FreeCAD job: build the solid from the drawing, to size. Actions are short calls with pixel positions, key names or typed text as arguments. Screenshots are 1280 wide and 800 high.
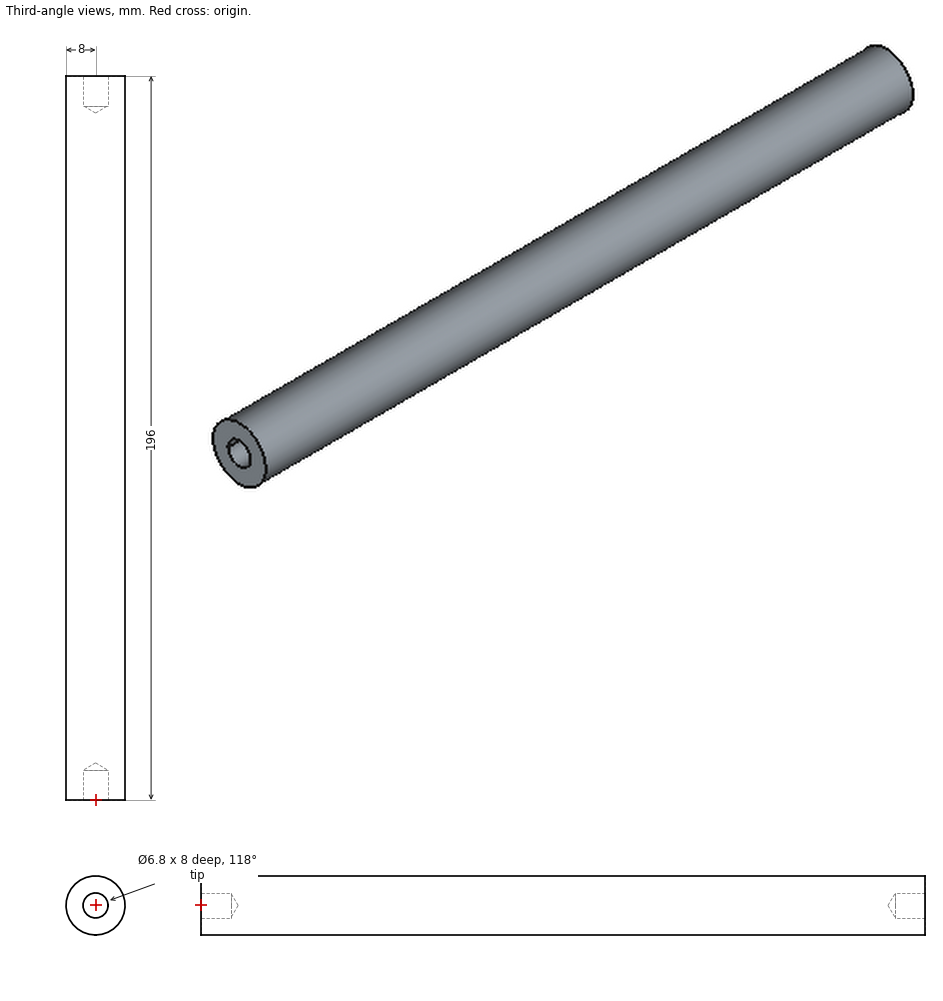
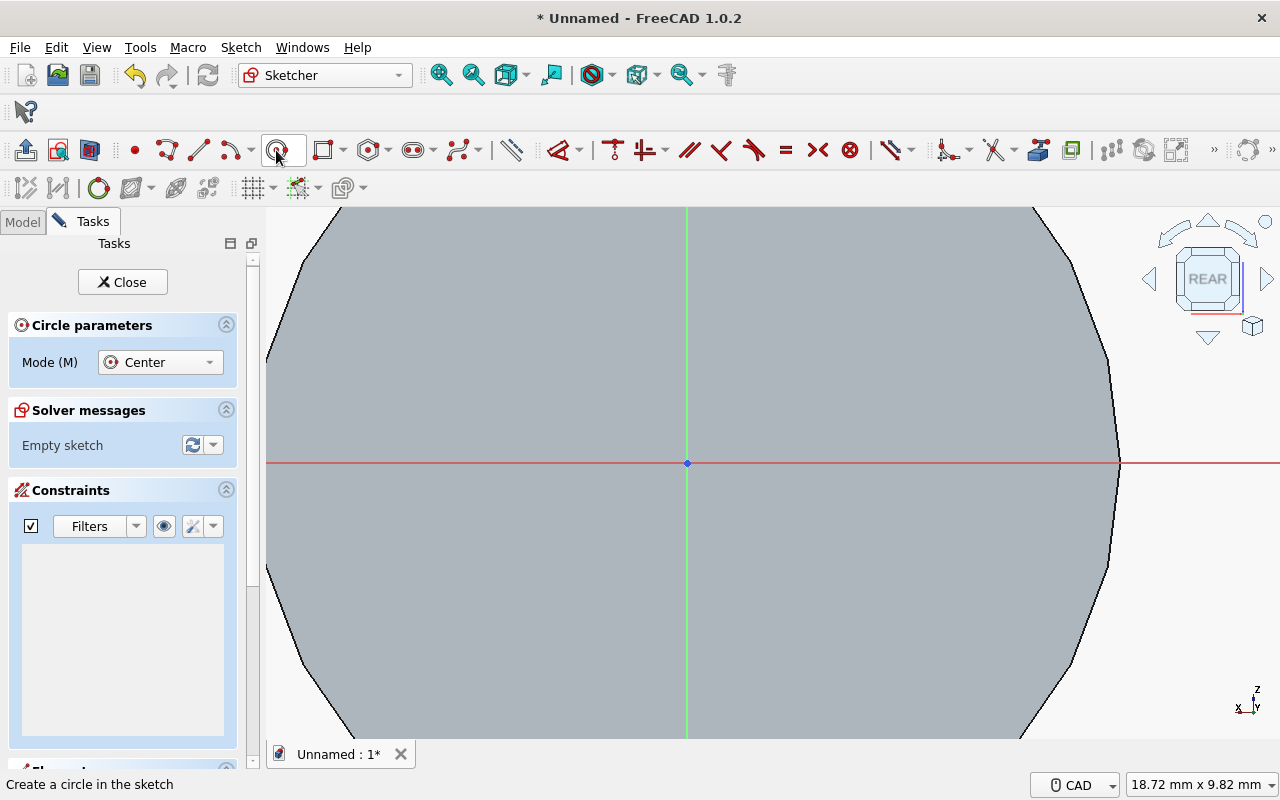
click(687, 463)
move(817, 333)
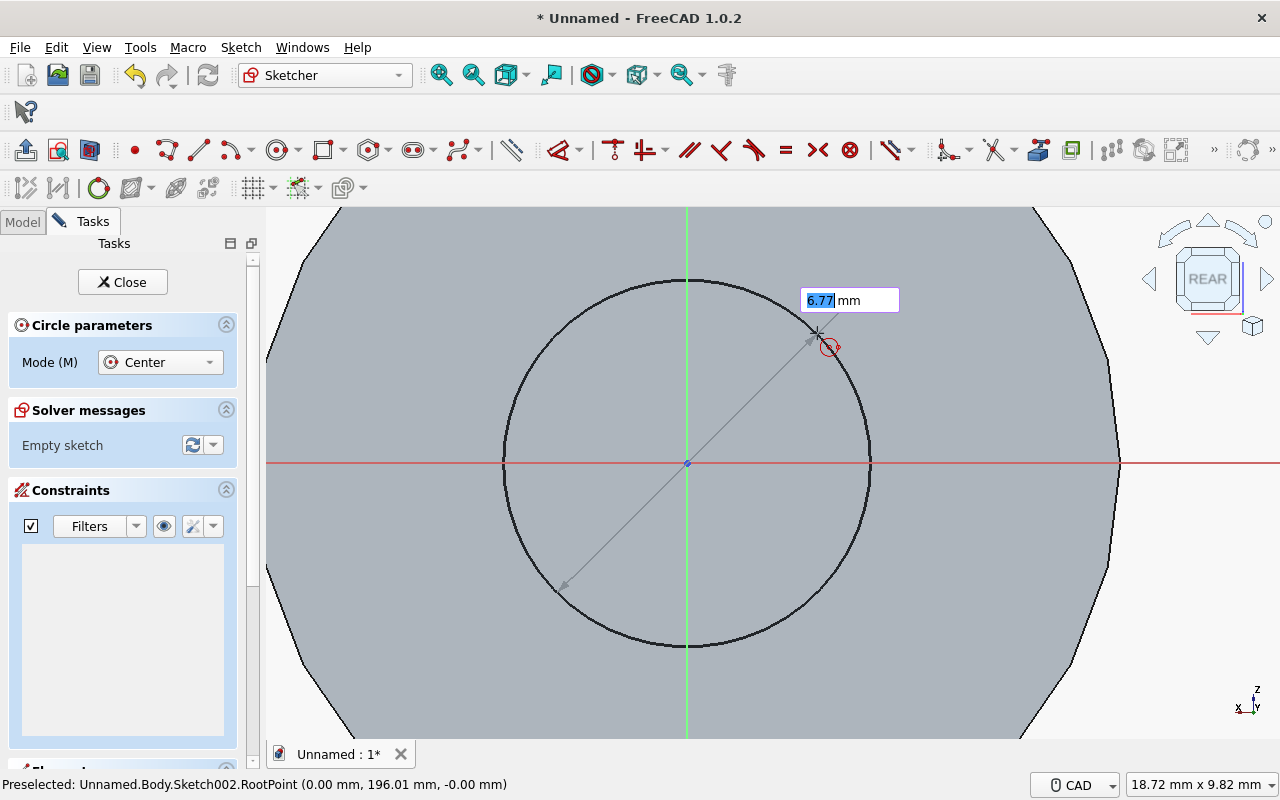
text(6.8)
key(Return)
key(Escape)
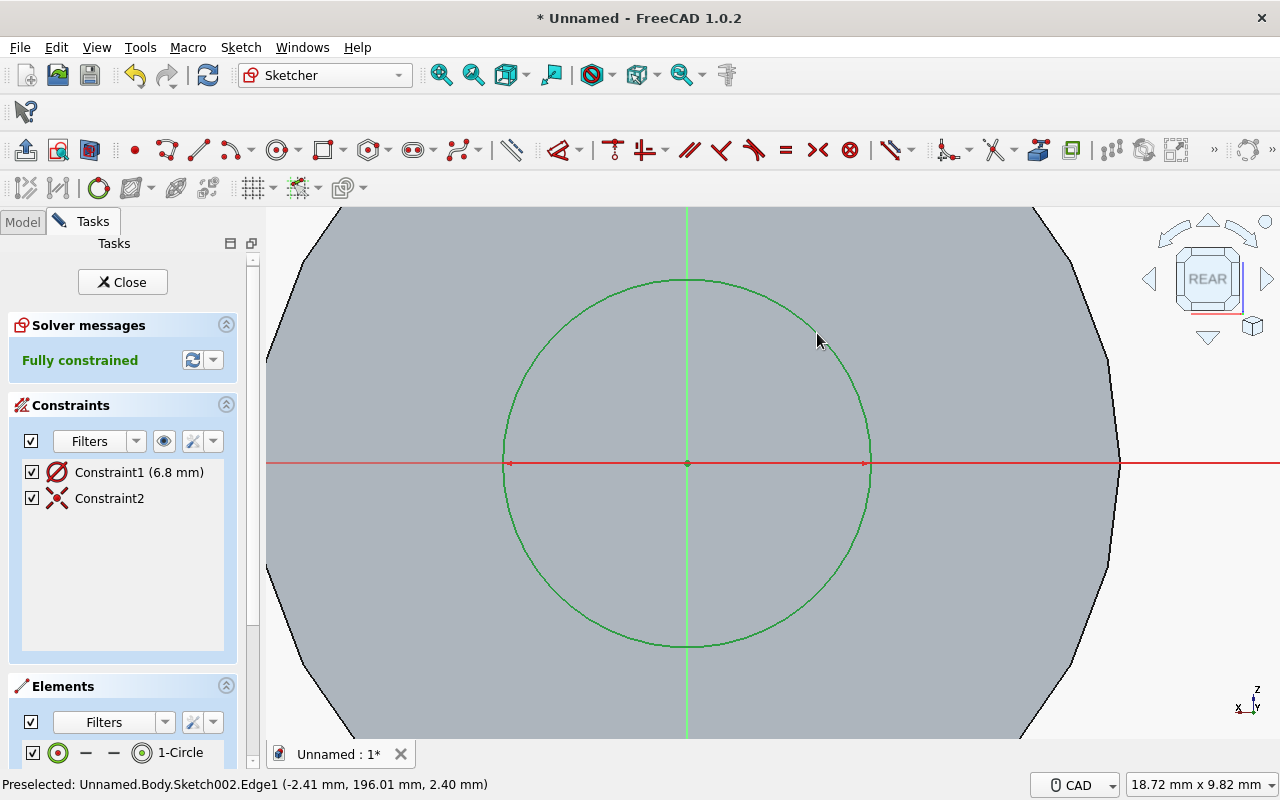
click(123, 282)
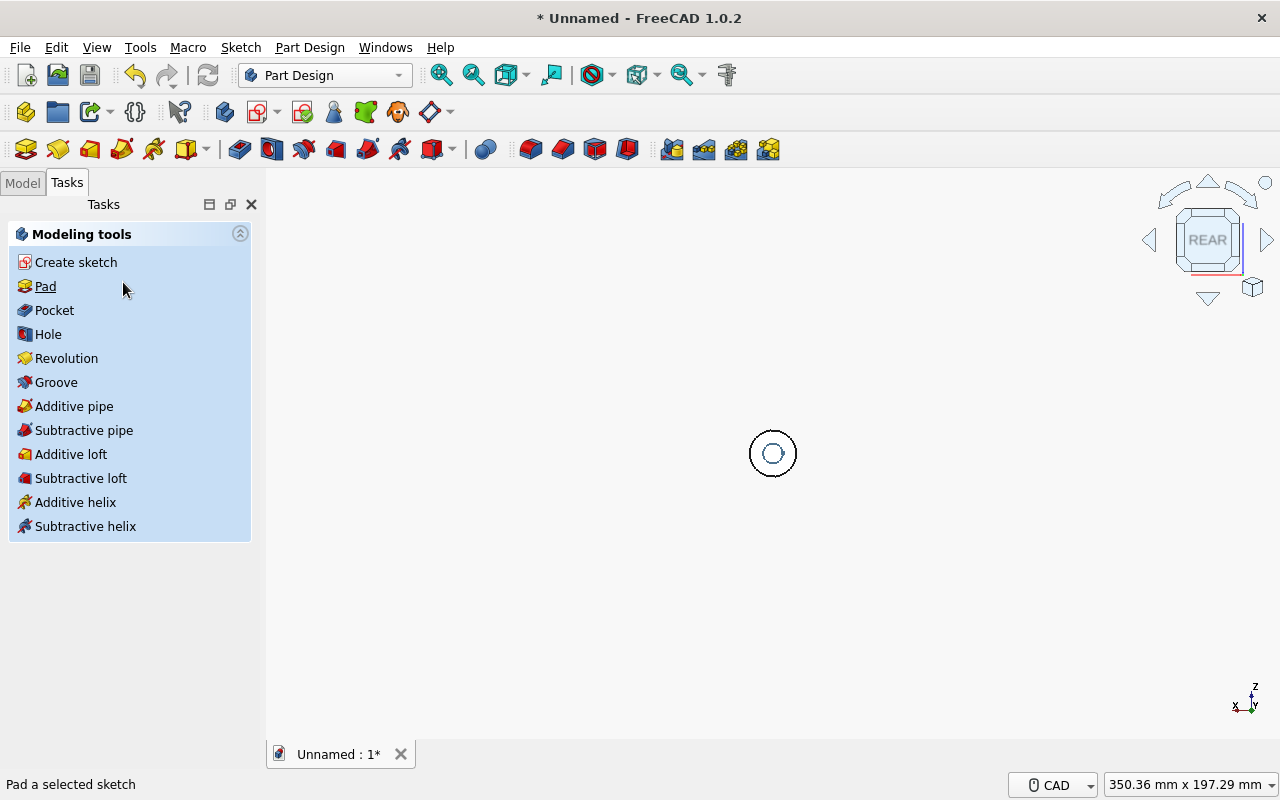
click(272, 150)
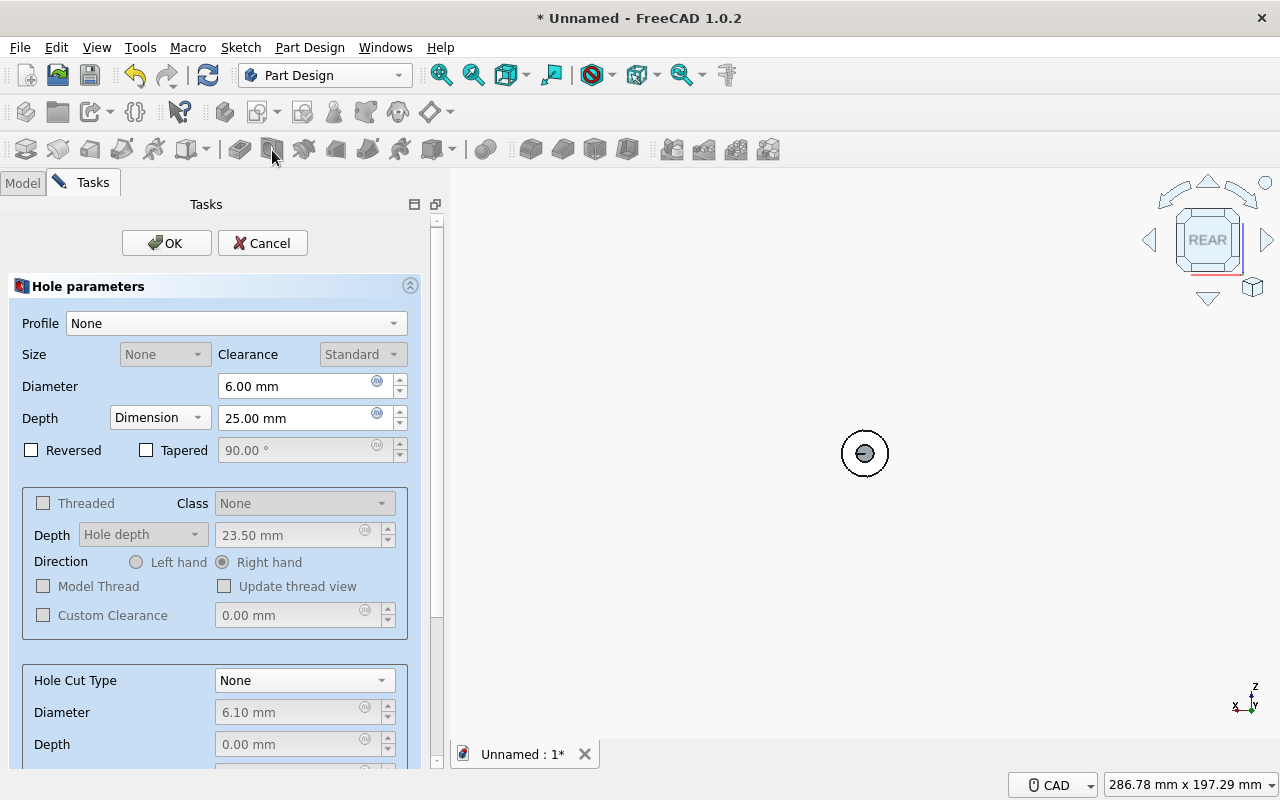
triple_click(305, 386)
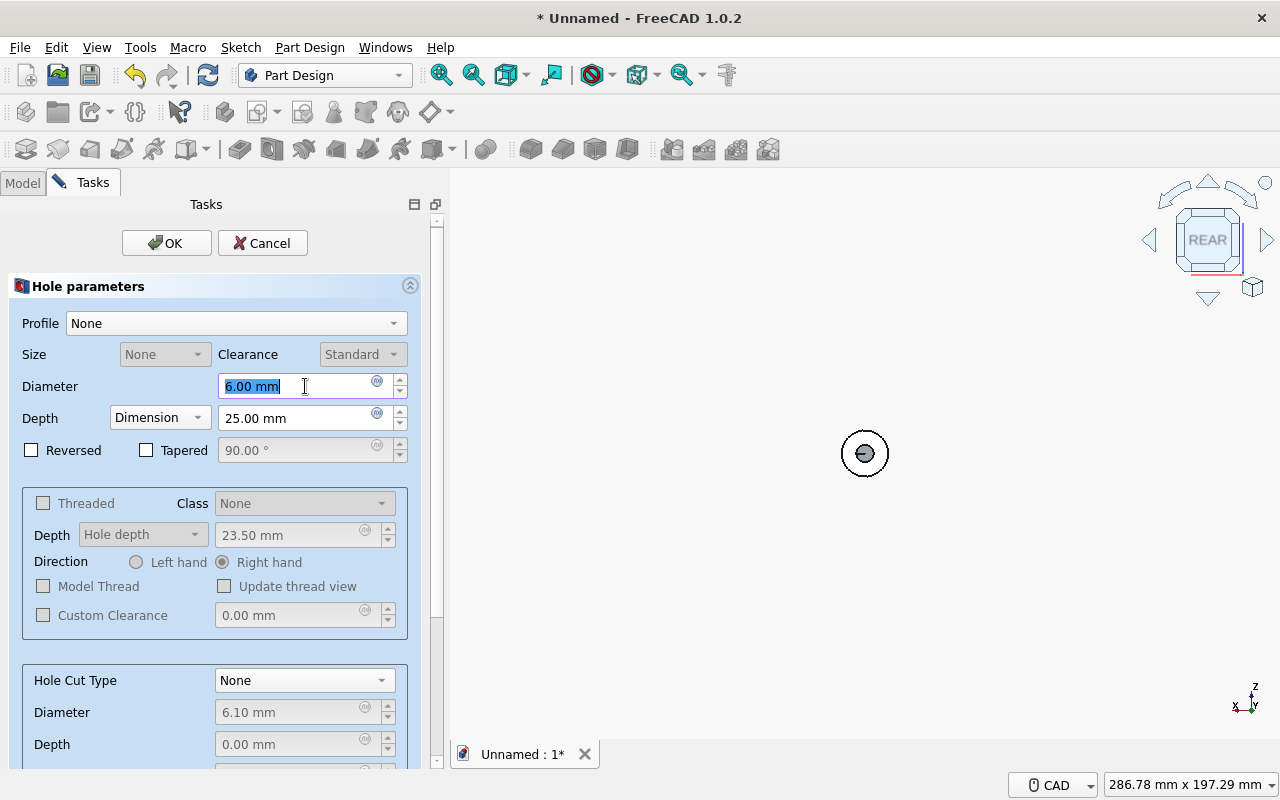
text(6.8)
key(Tab)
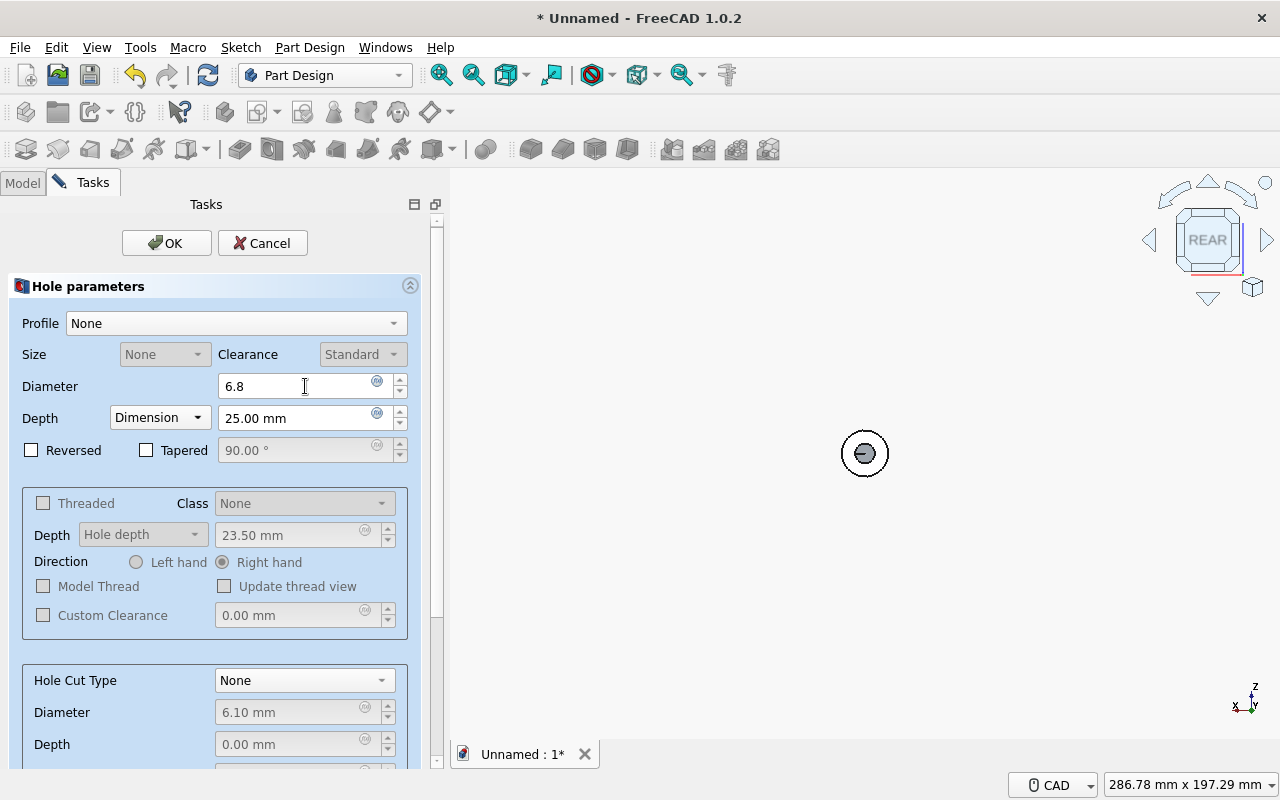
triple_click(305, 418)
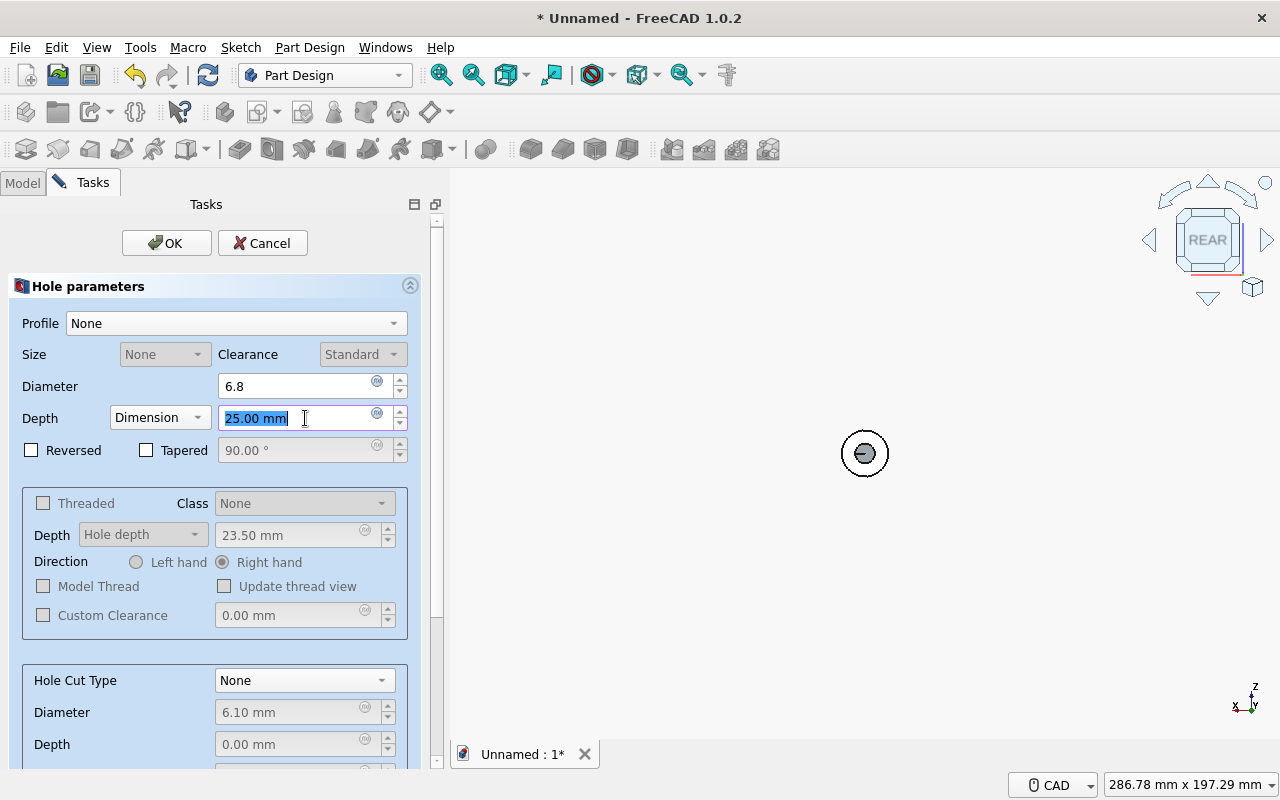
text(8)
key(Tab)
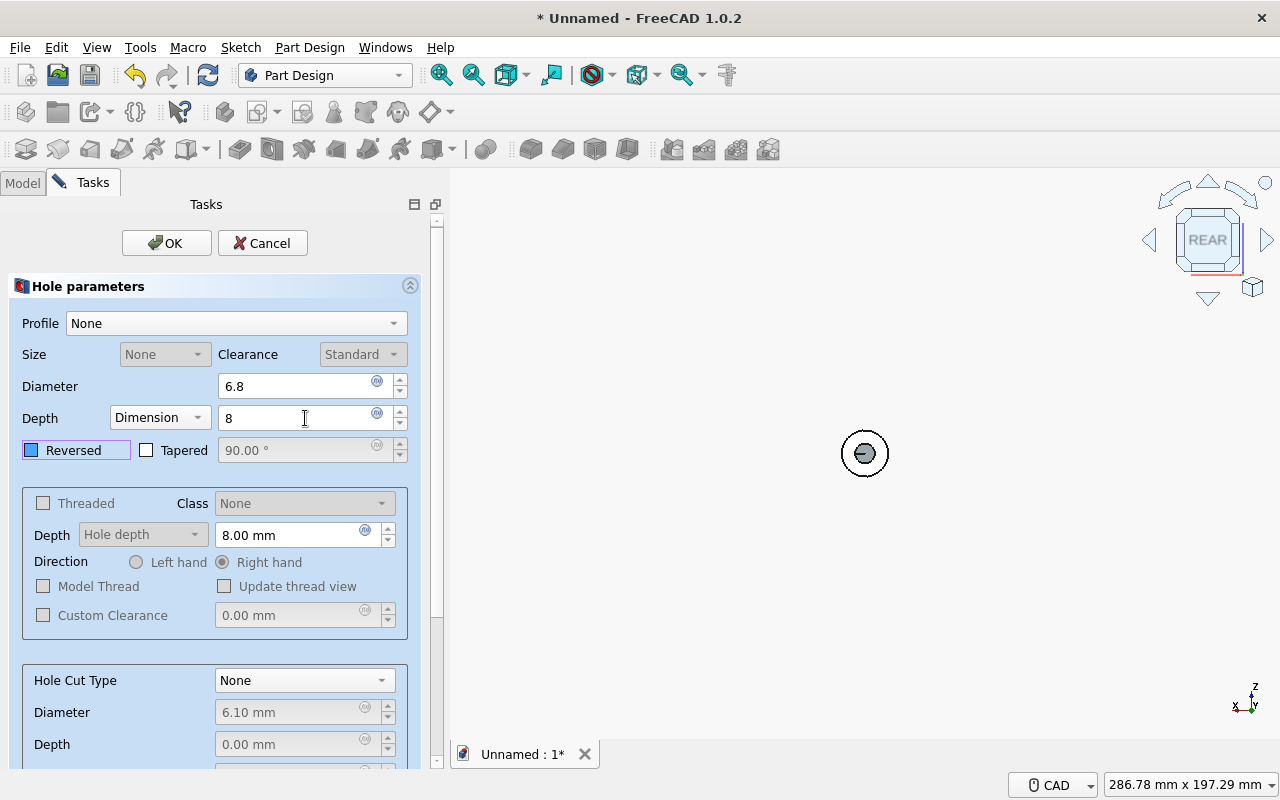
click(167, 243)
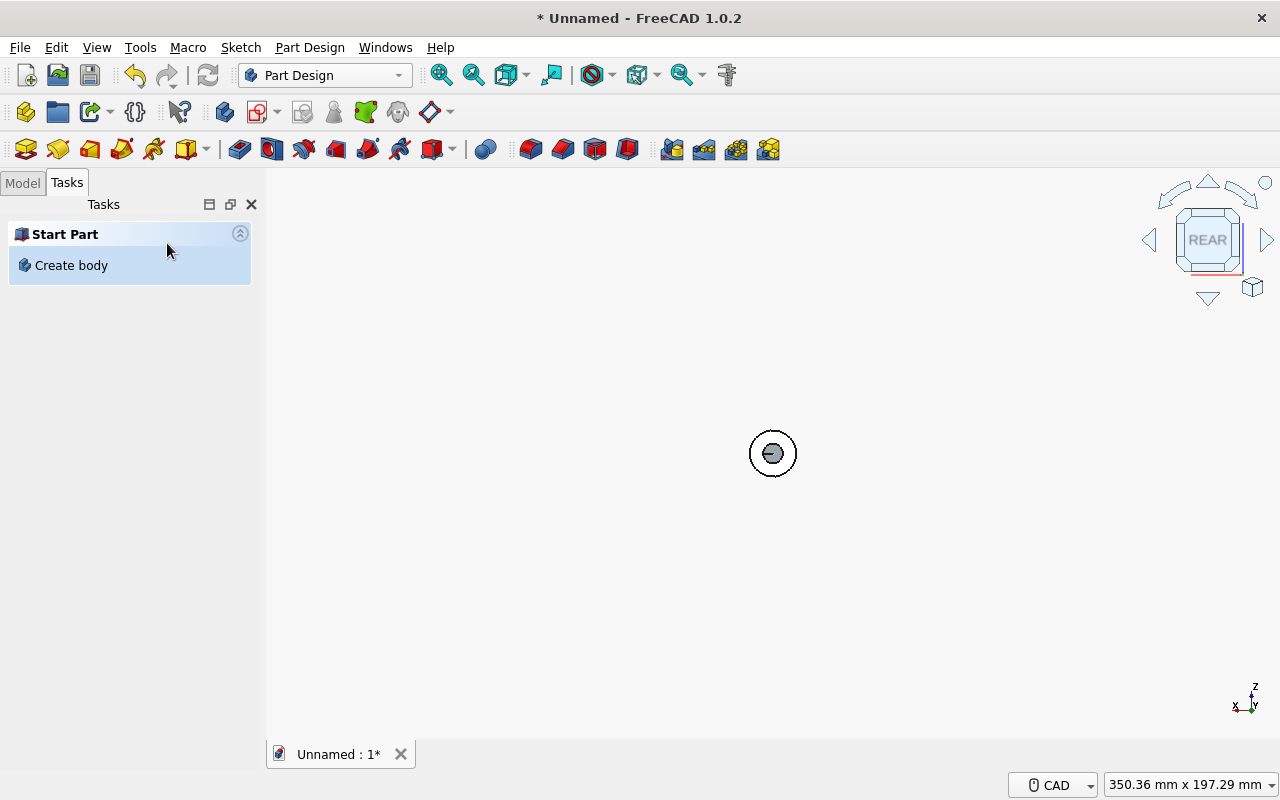
key(0)